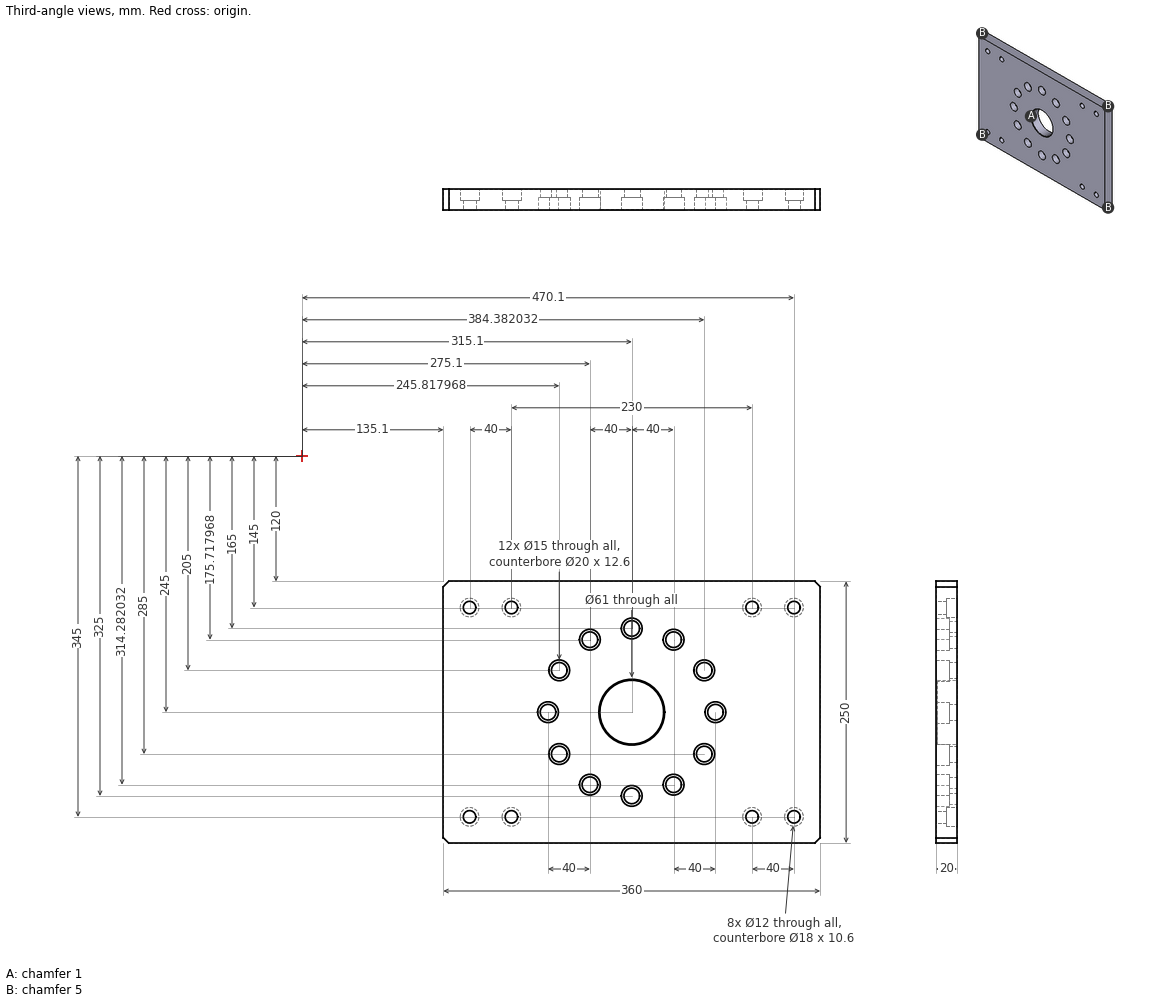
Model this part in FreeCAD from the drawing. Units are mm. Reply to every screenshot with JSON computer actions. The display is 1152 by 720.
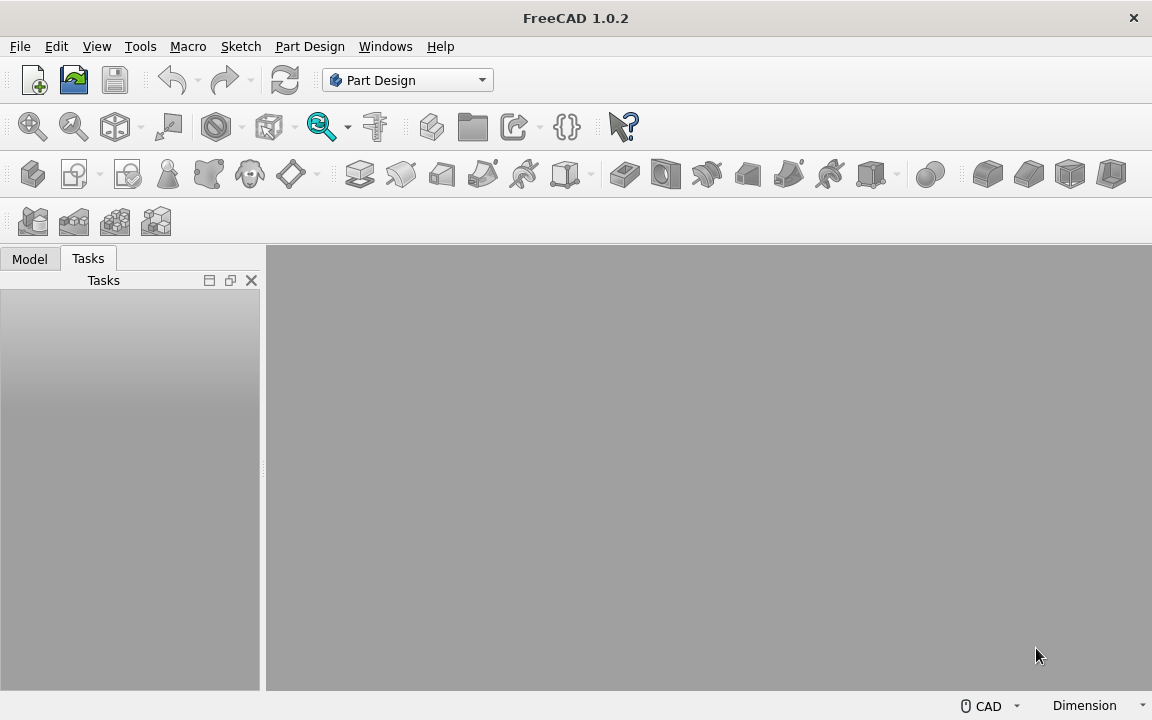
{"action": "left_click", "coordinate": [33, 80]}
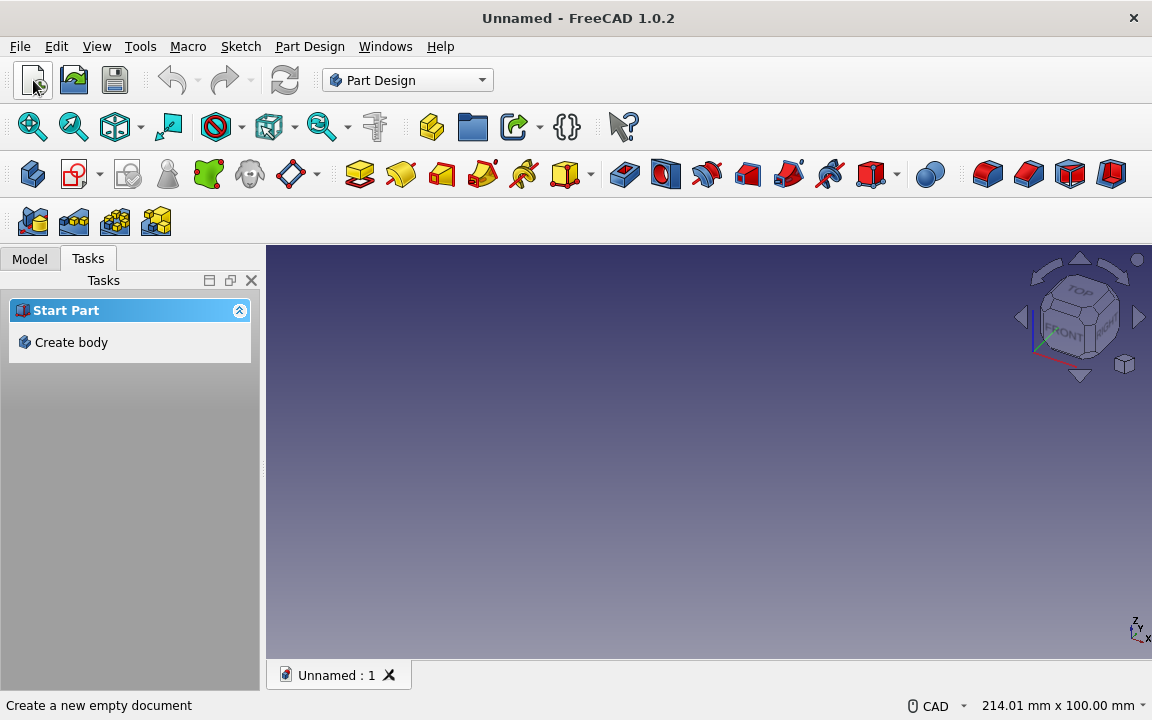
{"action": "left_click", "coordinate": [33, 174]}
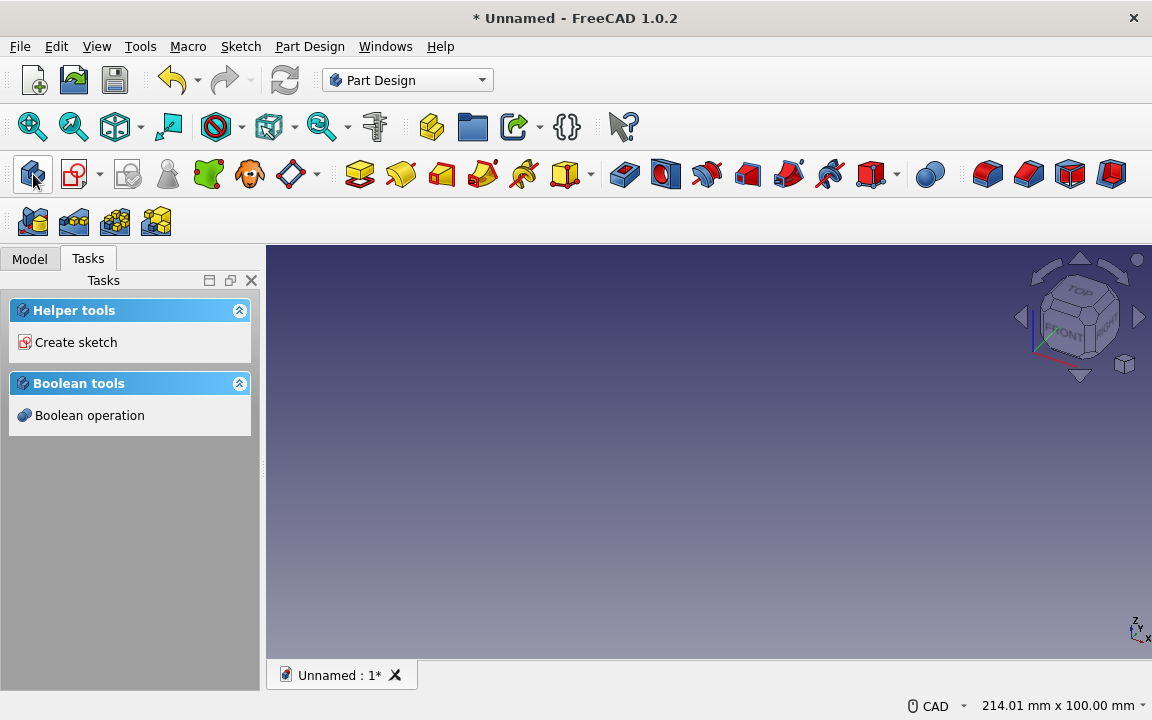
{"action": "left_click", "coordinate": [30, 258]}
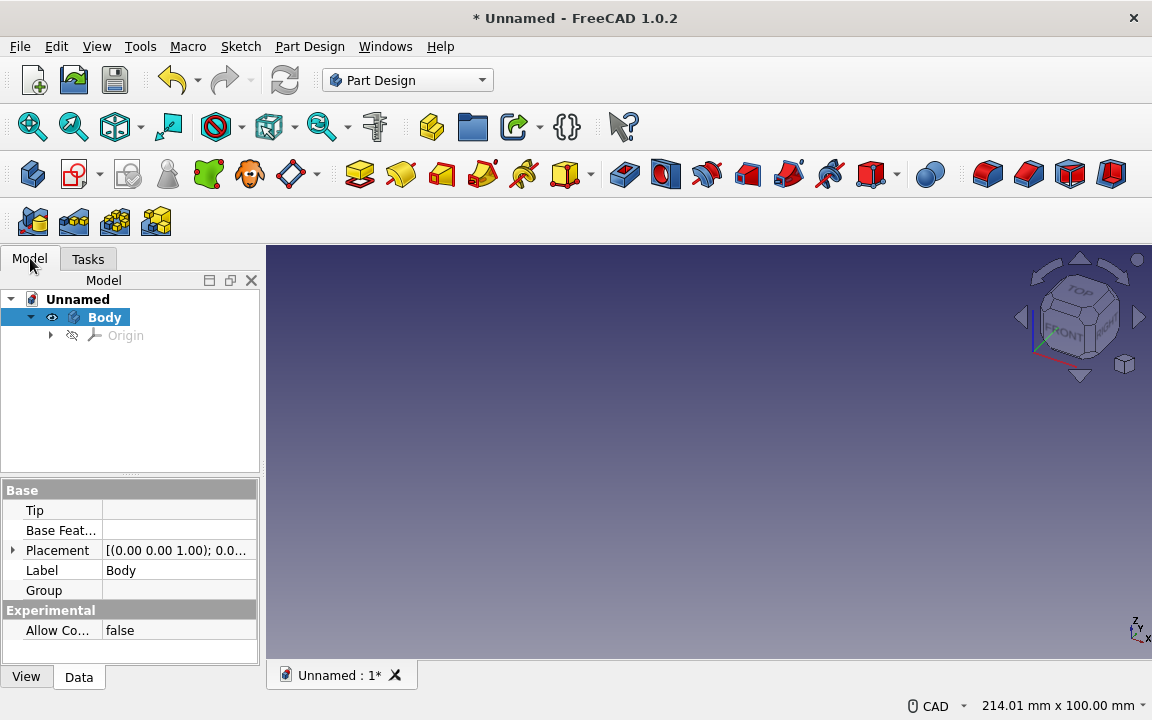
{"action": "left_click", "coordinate": [51, 335]}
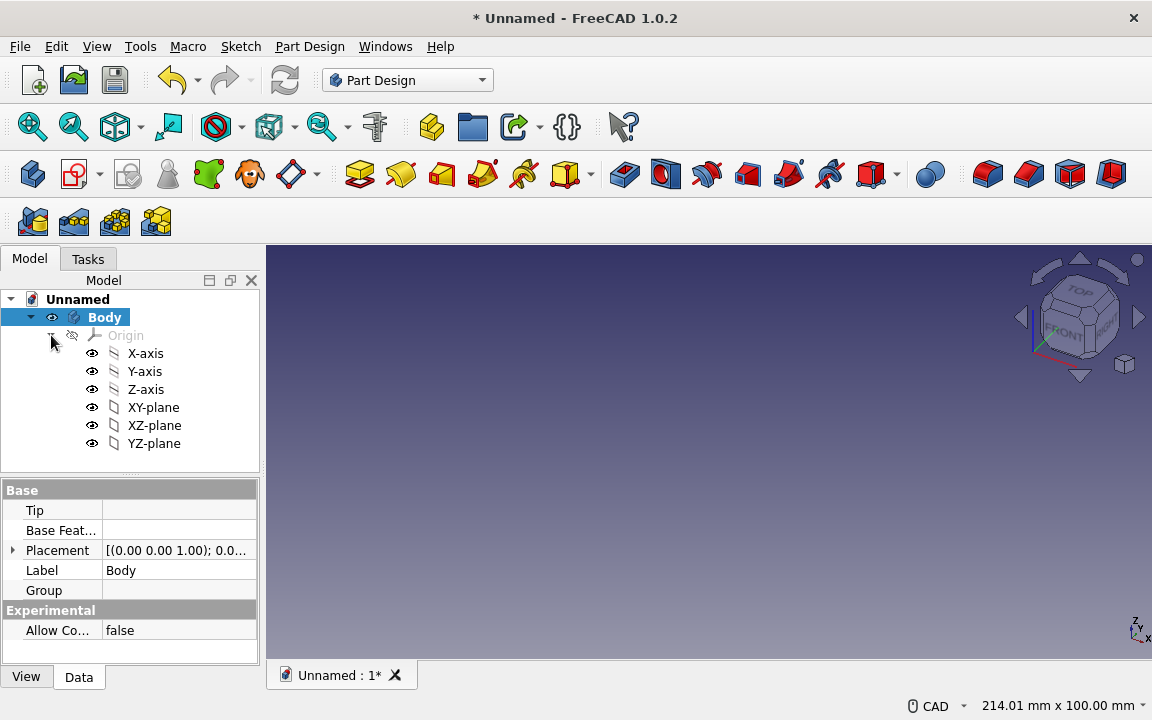
{"action": "left_click", "coordinate": [137, 425]}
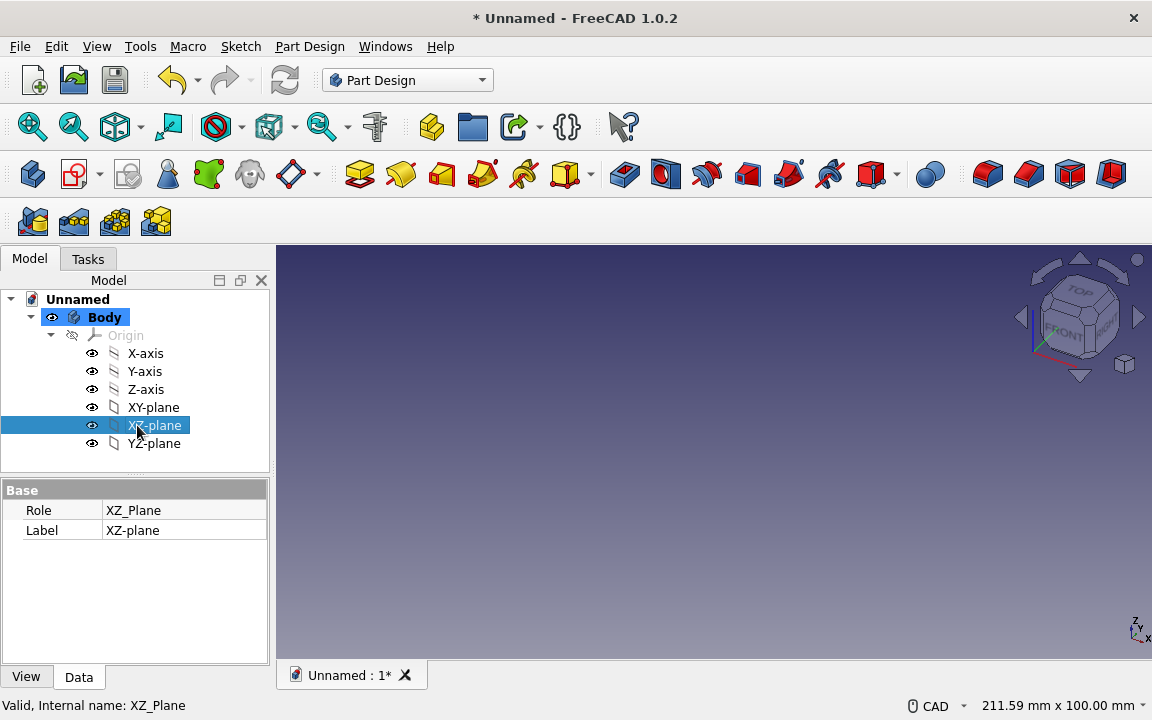
{"action": "left_click", "coordinate": [290, 174]}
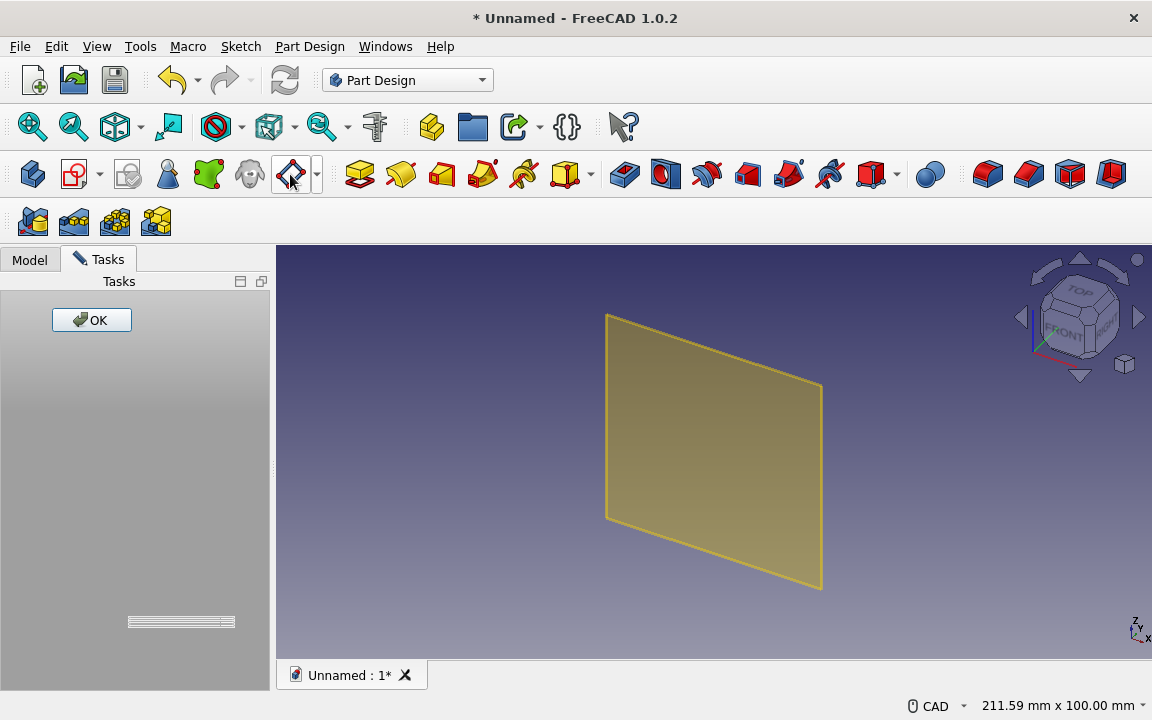
{"action": "scroll", "coordinate": [346, 490], "scroll_direction": "down", "scroll_amount": 4}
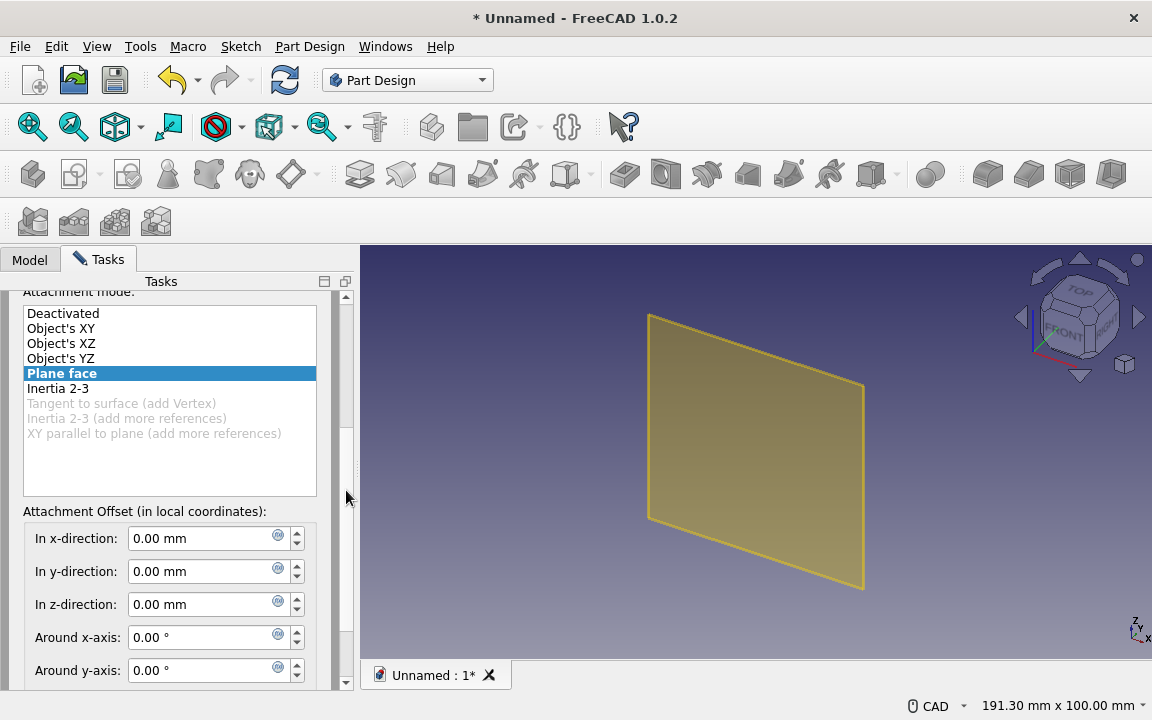
{"action": "triple_click", "coordinate": [210, 604]}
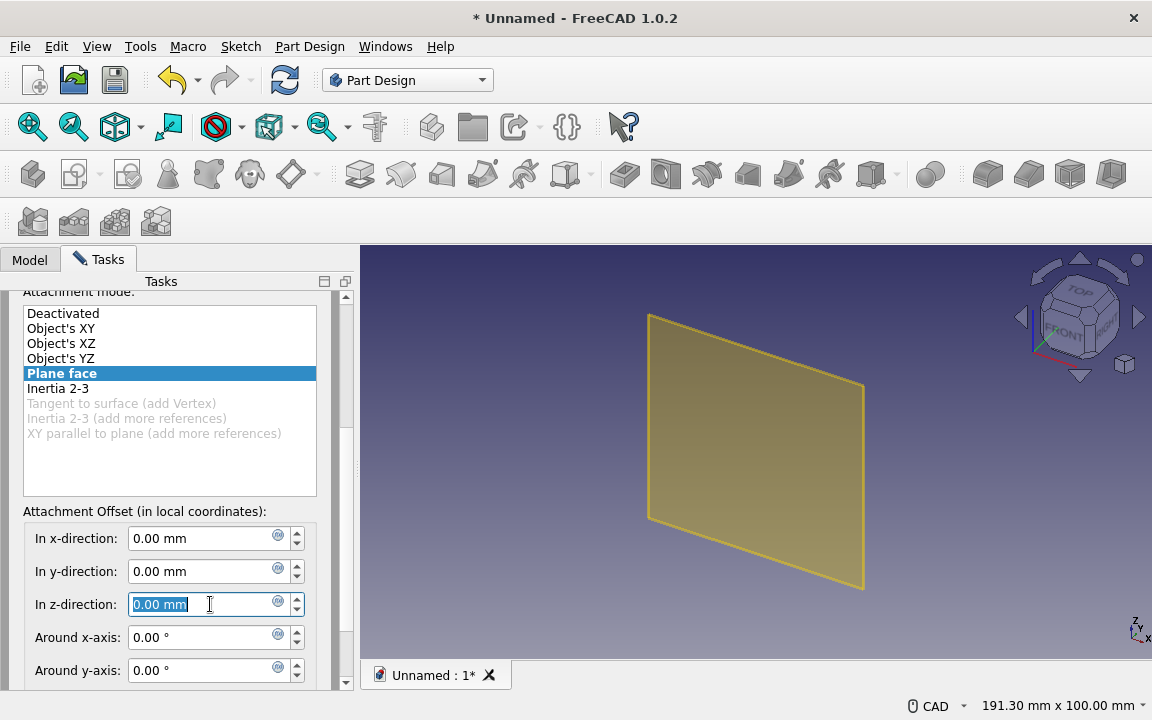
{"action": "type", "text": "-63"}
{"action": "key", "text": "Tab"}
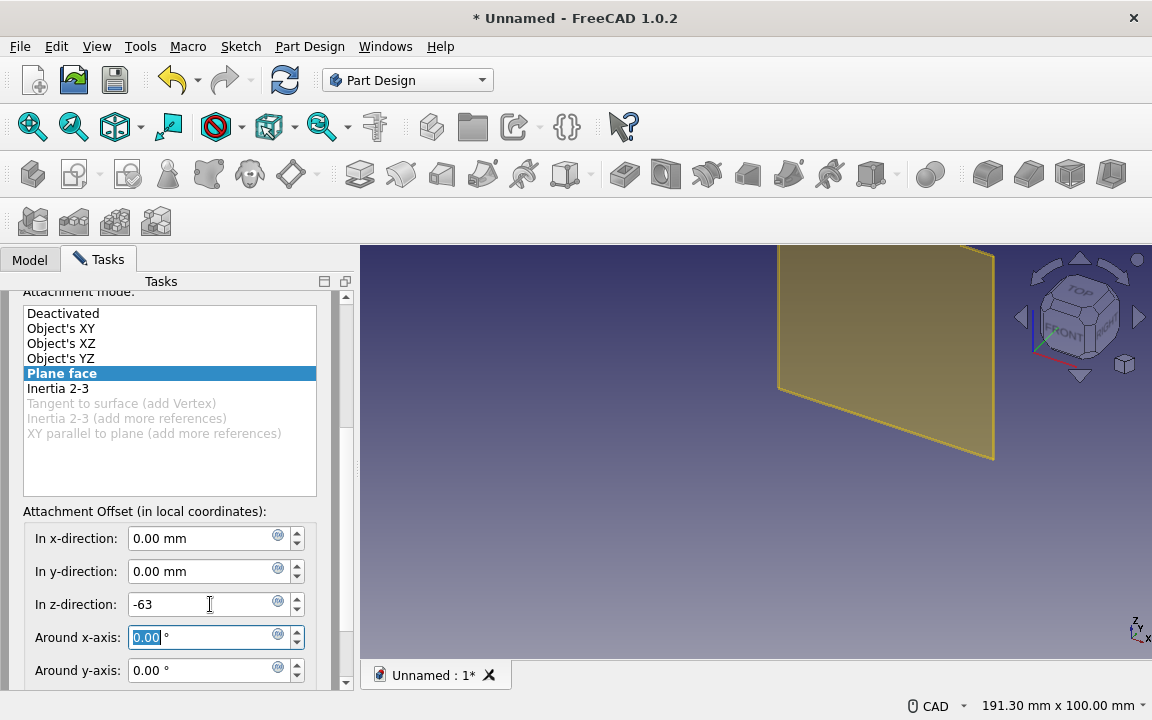
{"action": "scroll", "coordinate": [346, 490], "scroll_direction": "up", "scroll_amount": 5}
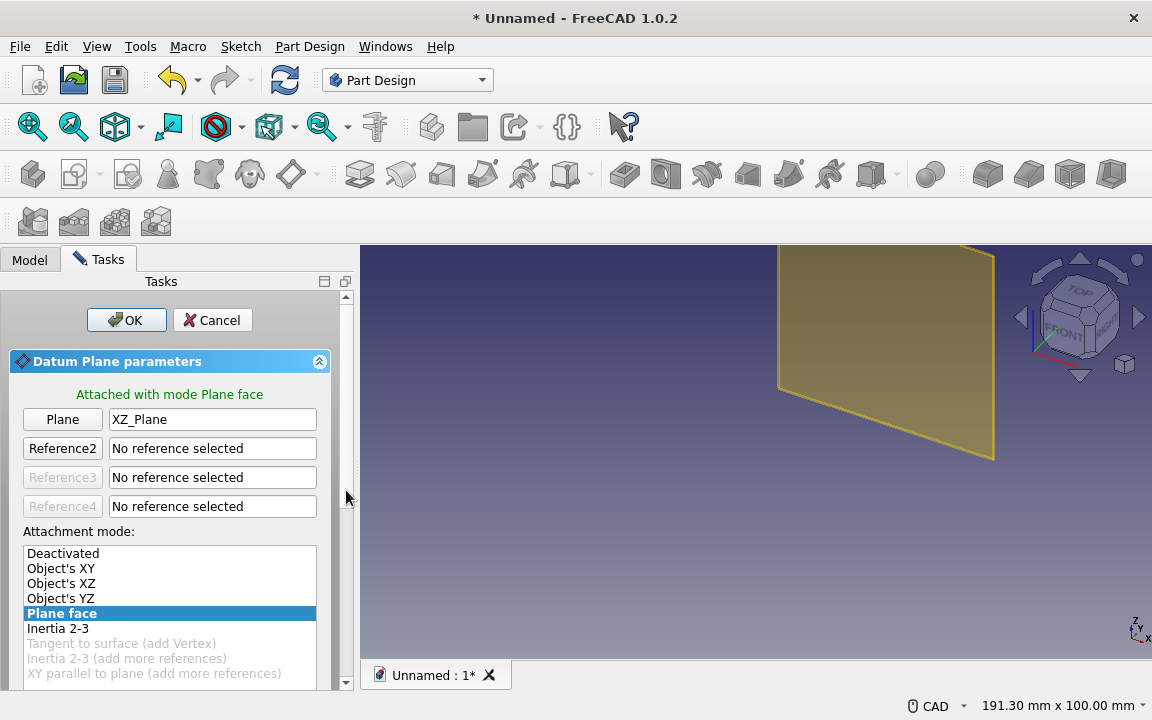
{"action": "left_click", "coordinate": [127, 320]}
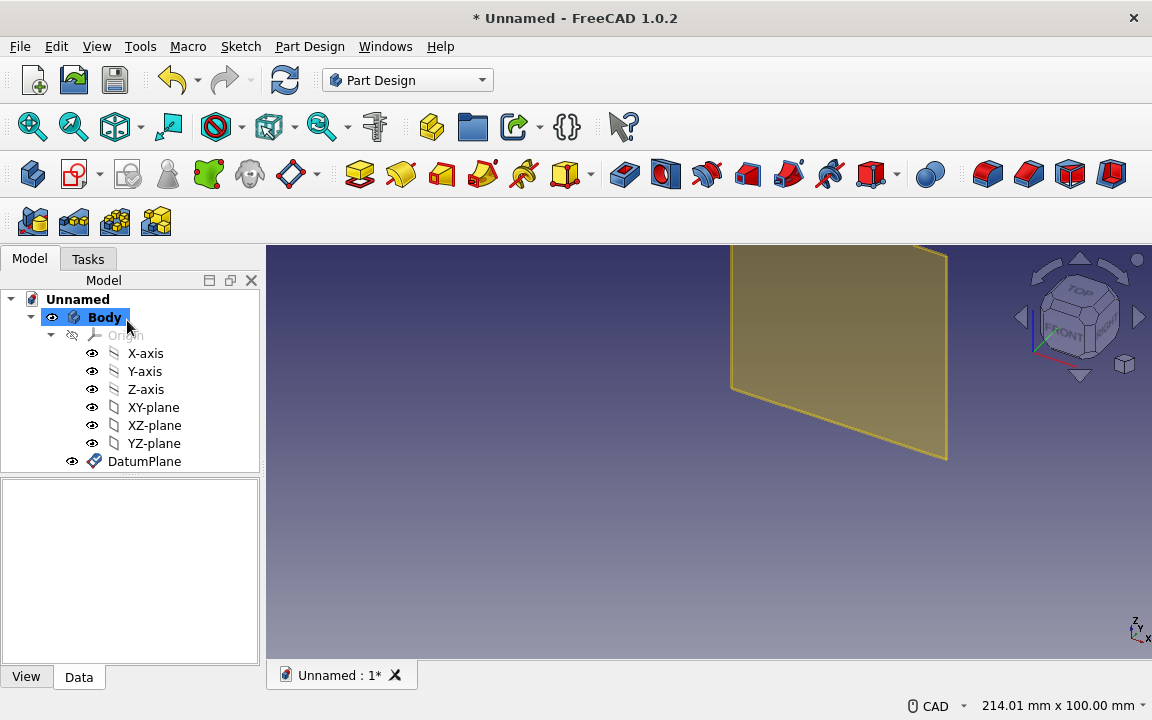
{"action": "left_click", "coordinate": [117, 461]}